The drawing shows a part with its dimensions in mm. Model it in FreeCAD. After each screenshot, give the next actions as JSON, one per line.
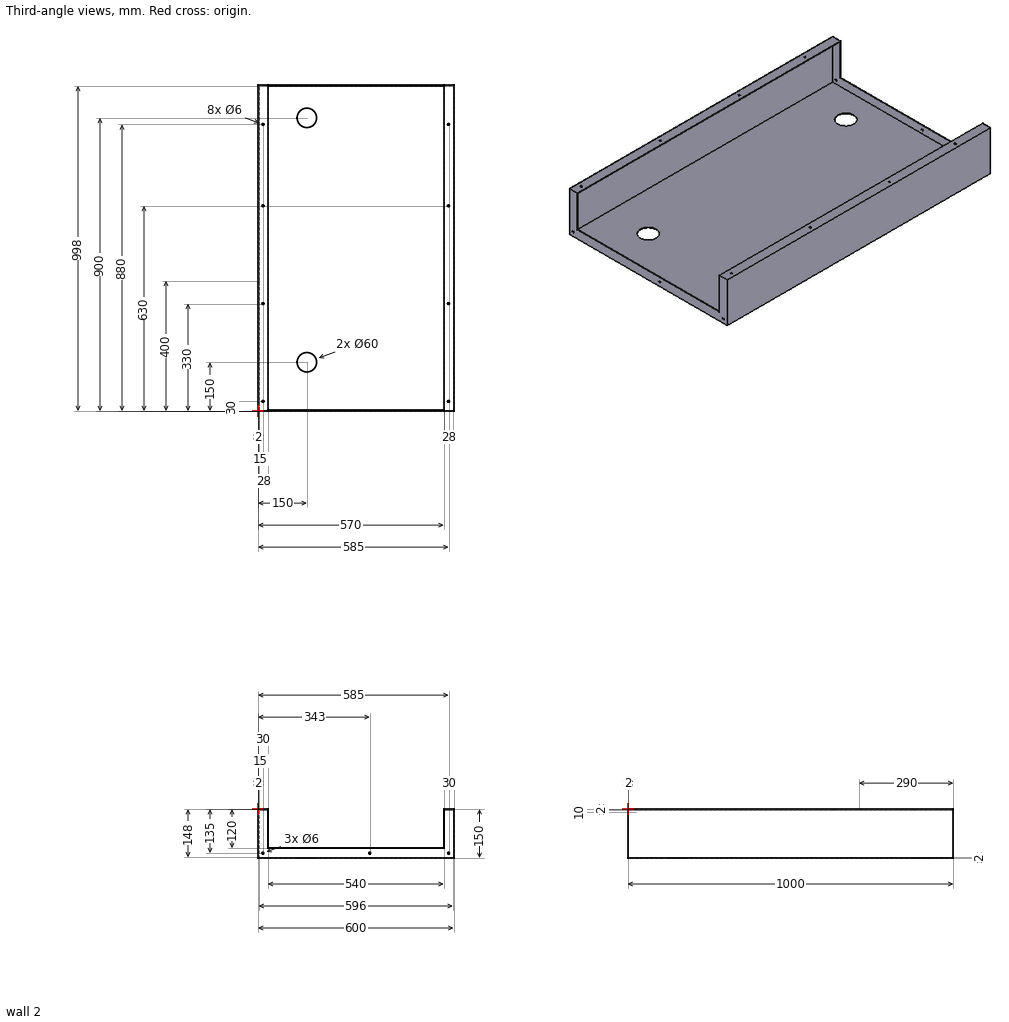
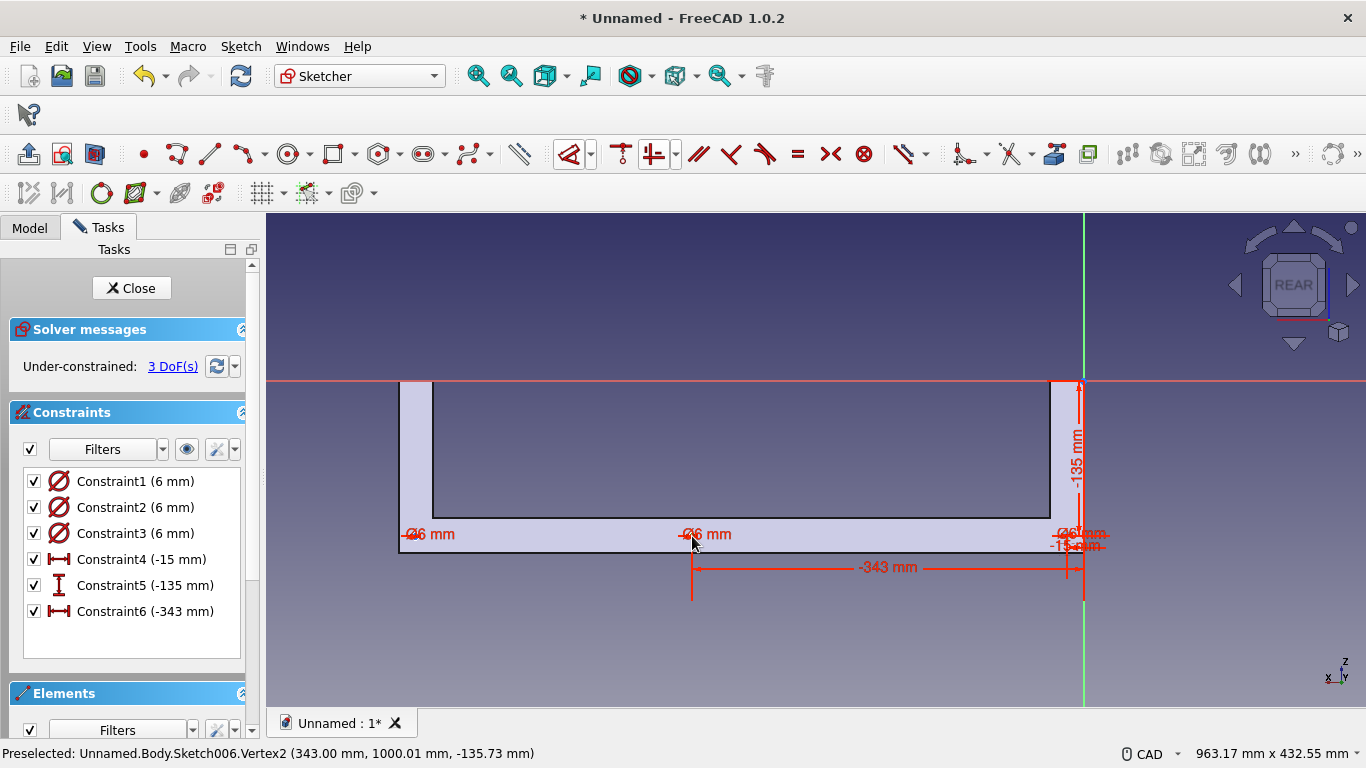
{"action": "key", "text": "i"}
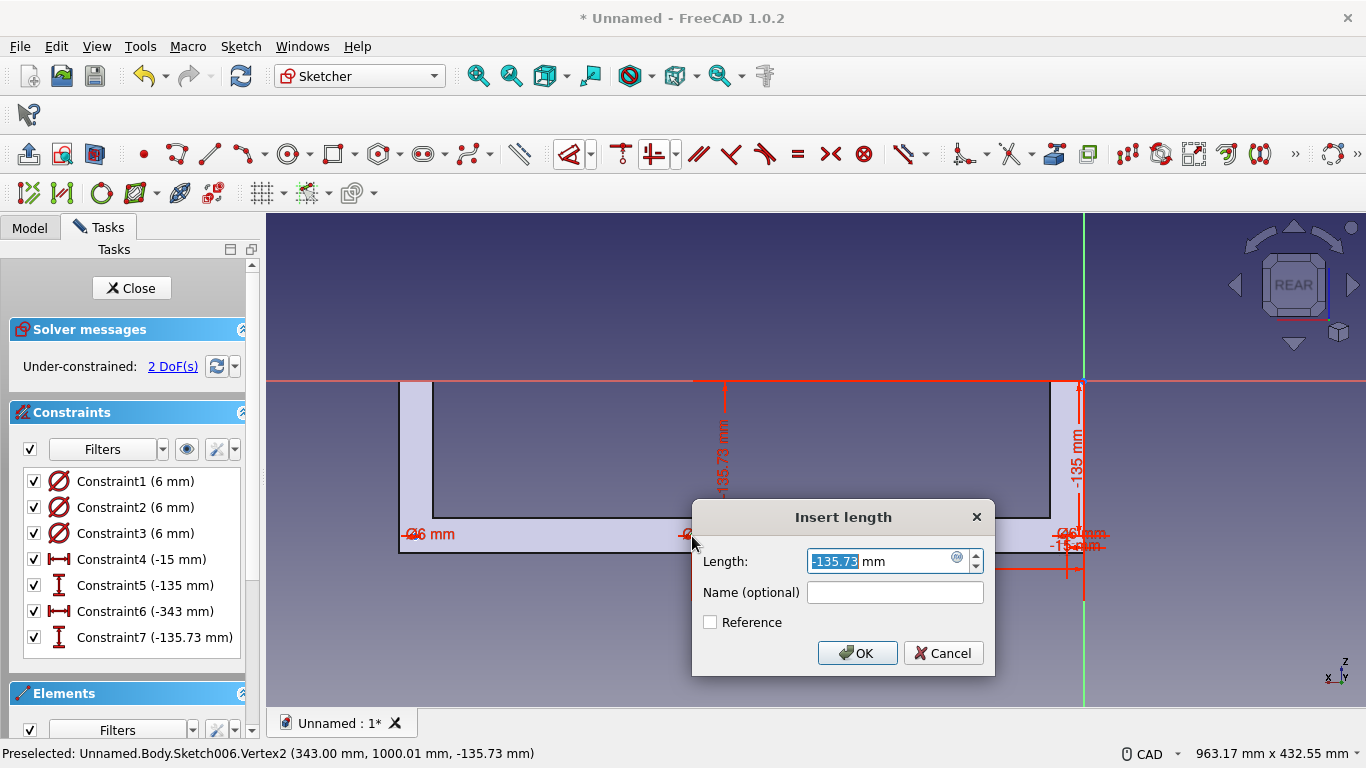
{"action": "type", "text": "-135"}
{"action": "key", "text": "Return"}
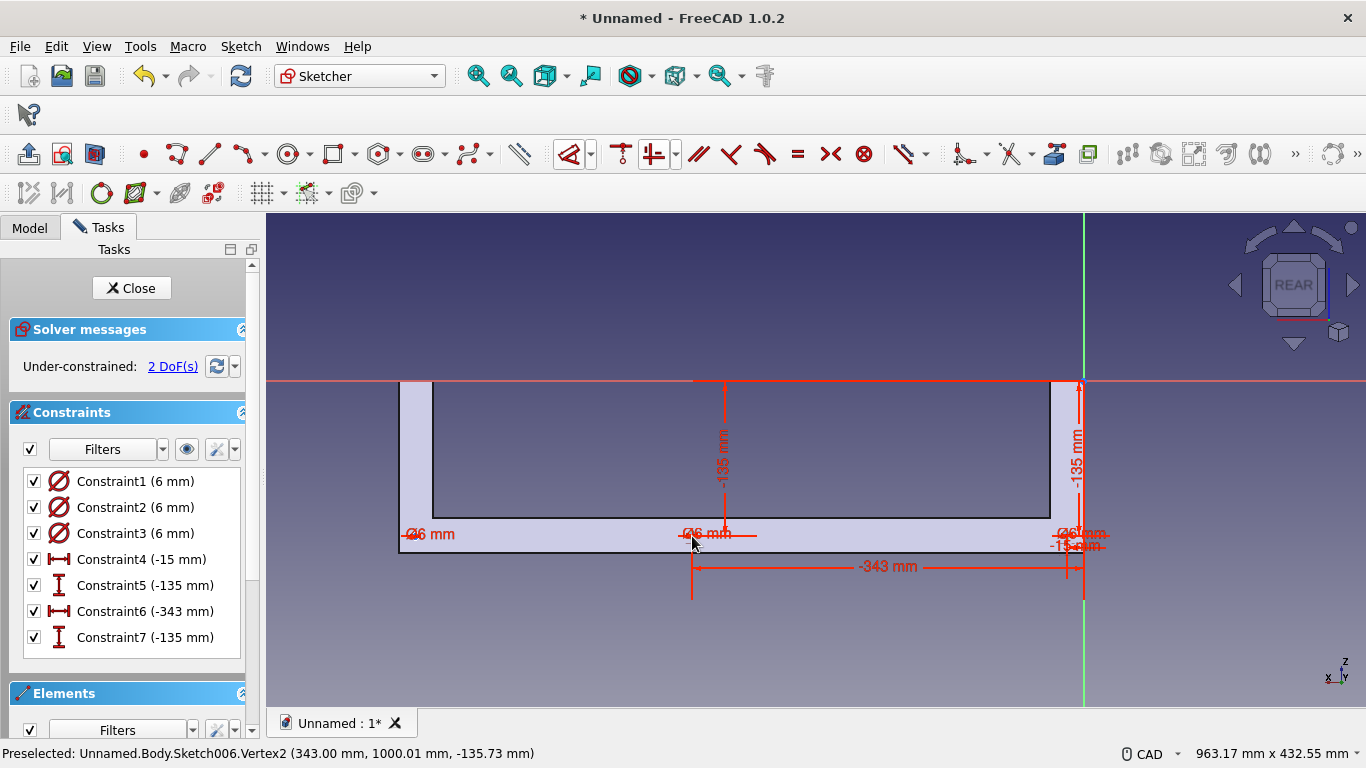
{"action": "left_click", "coordinate": [416, 536]}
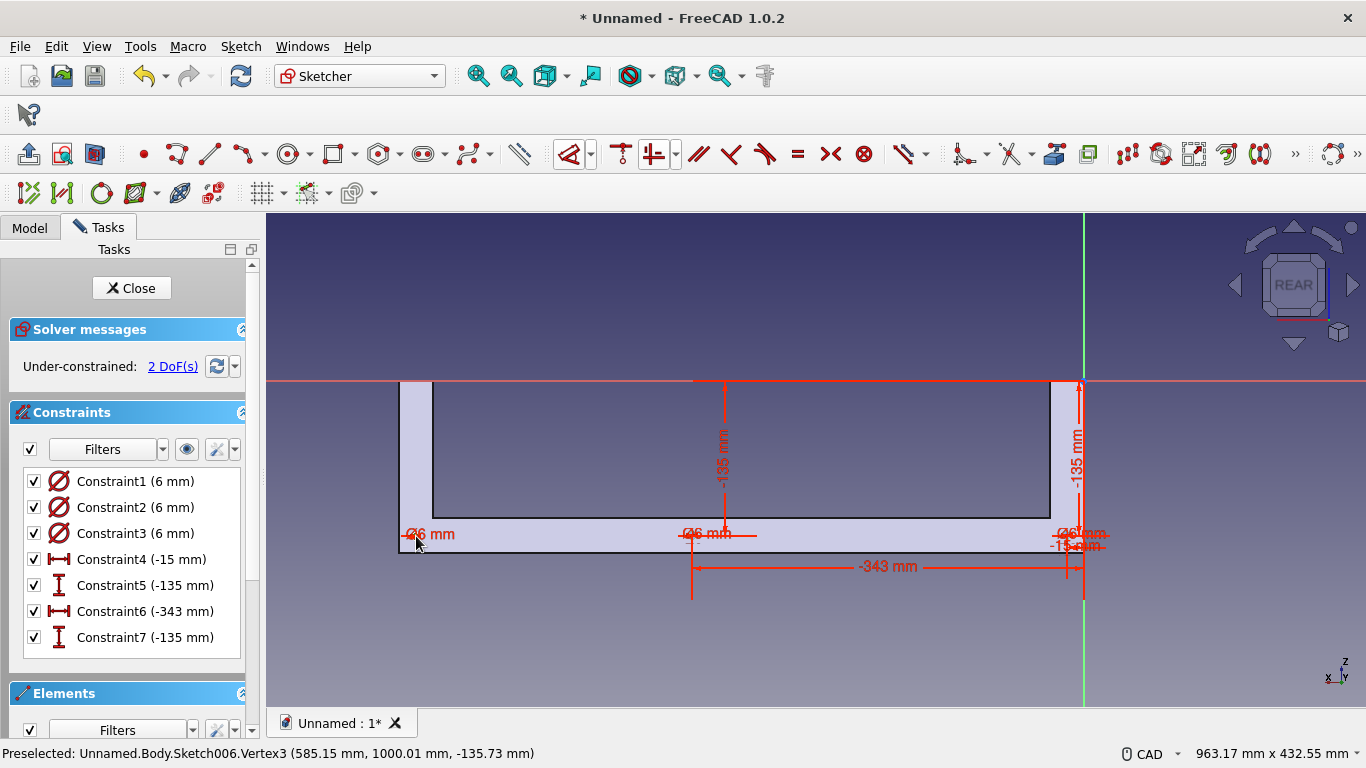
{"action": "left_click", "coordinate": [590, 154]}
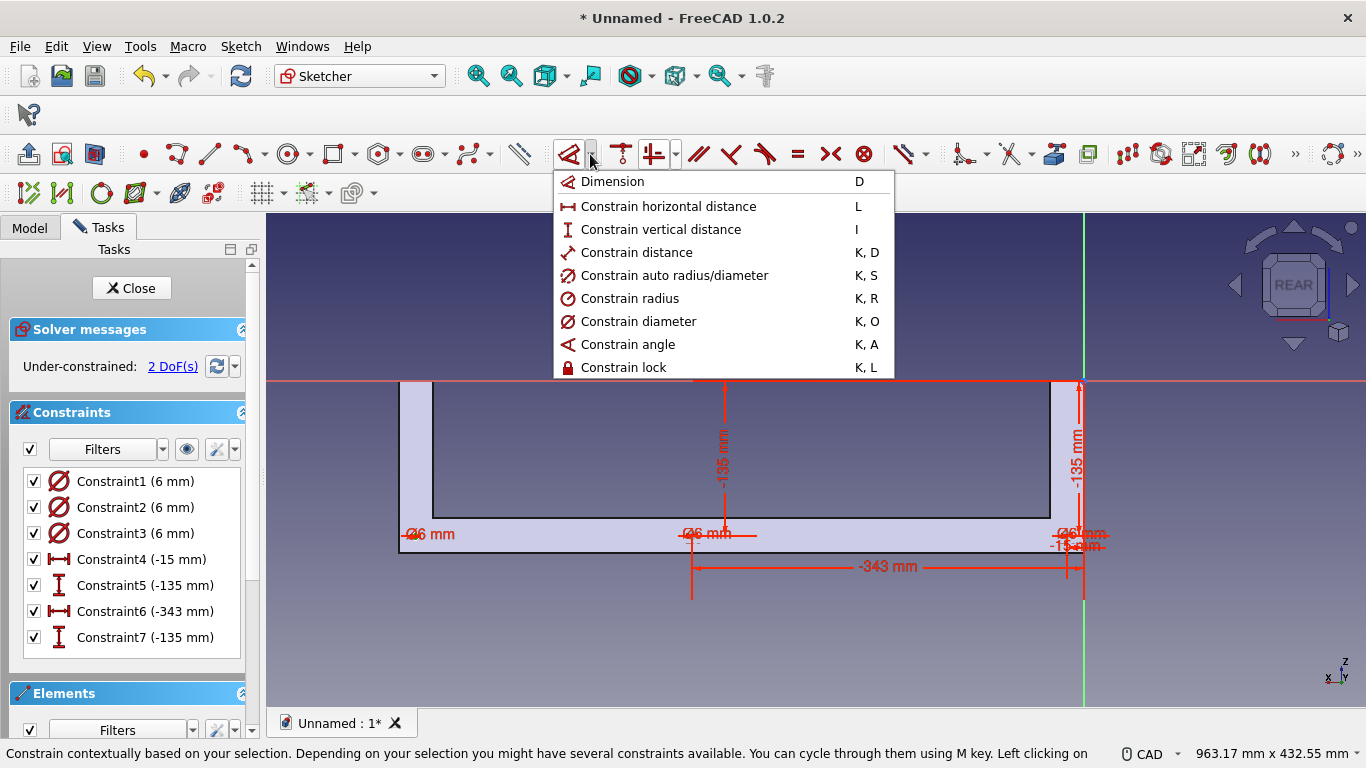
{"action": "left_click", "coordinate": [724, 206]}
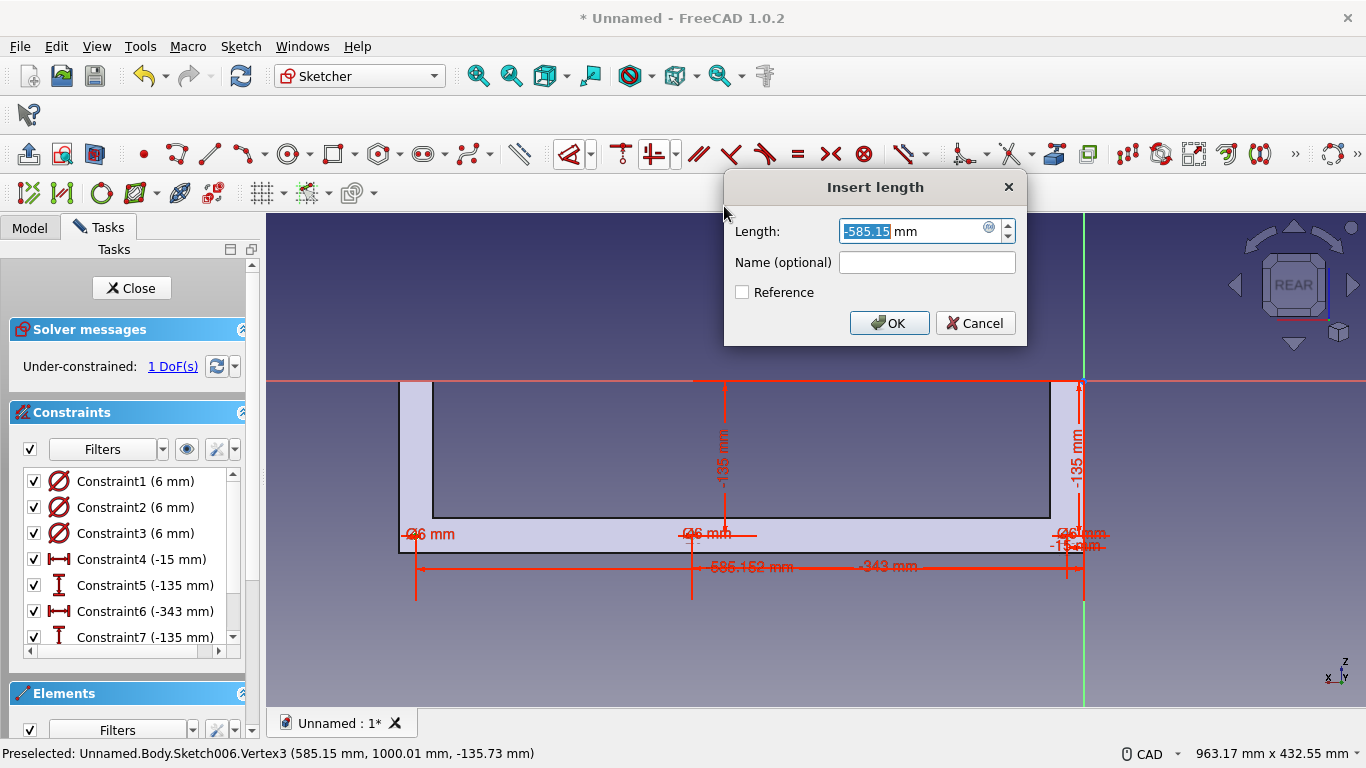
{"action": "type", "text": "-585"}
{"action": "key", "text": "Return"}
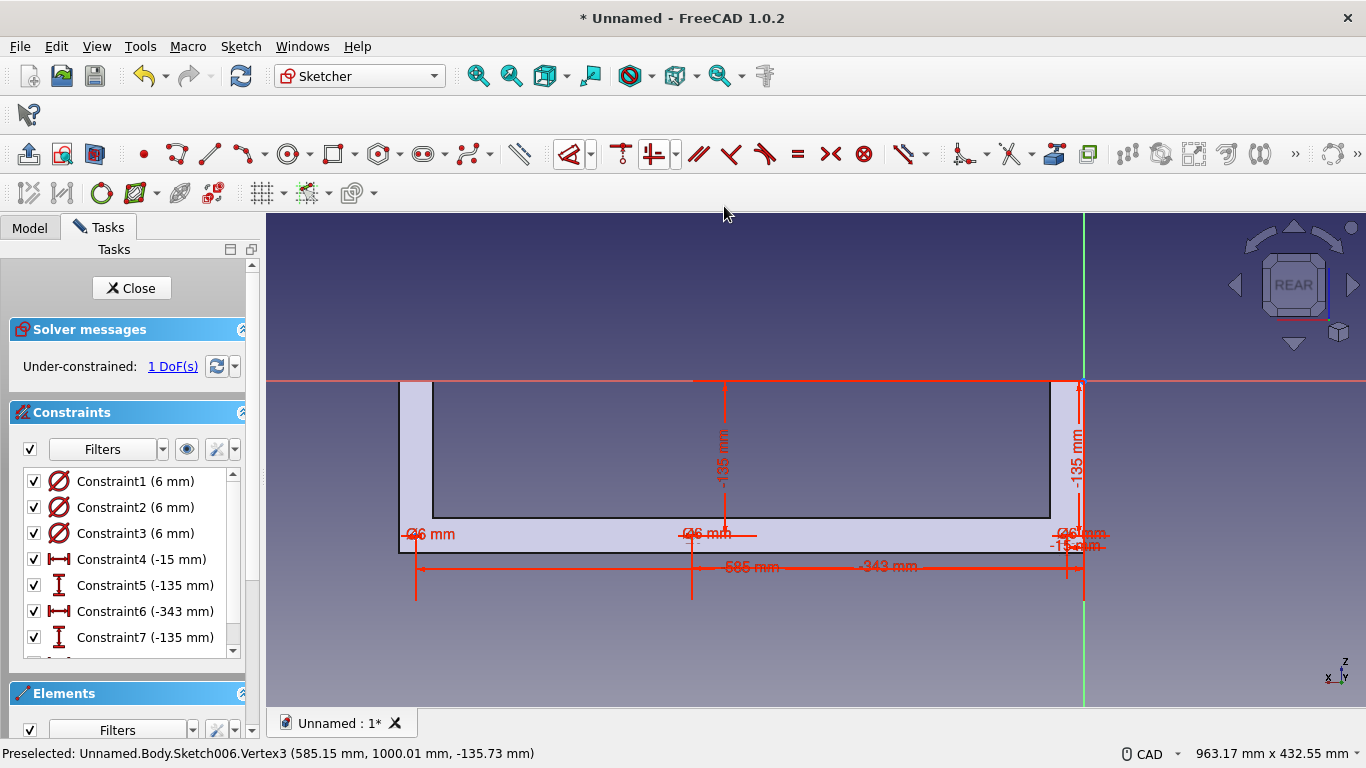
{"action": "left_click", "coordinate": [416, 536]}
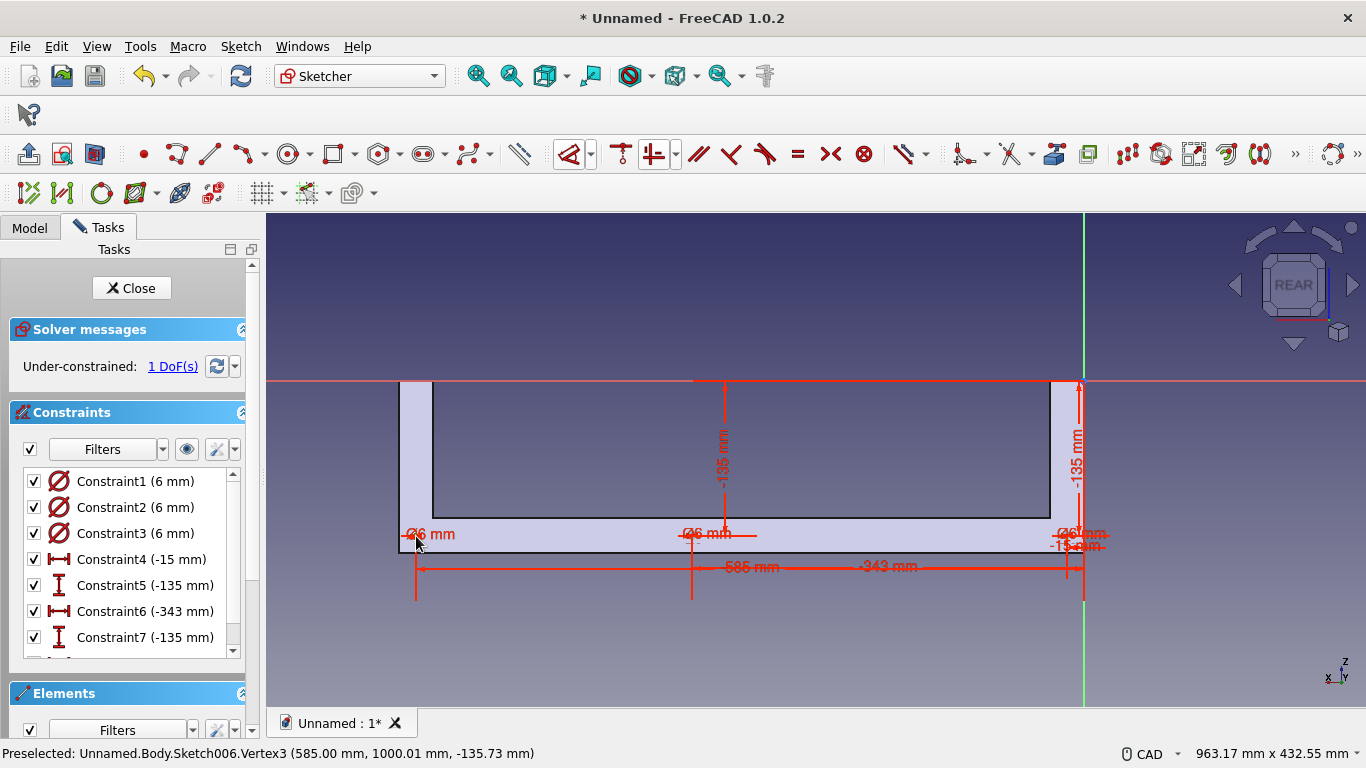
{"action": "left_click", "coordinate": [590, 154]}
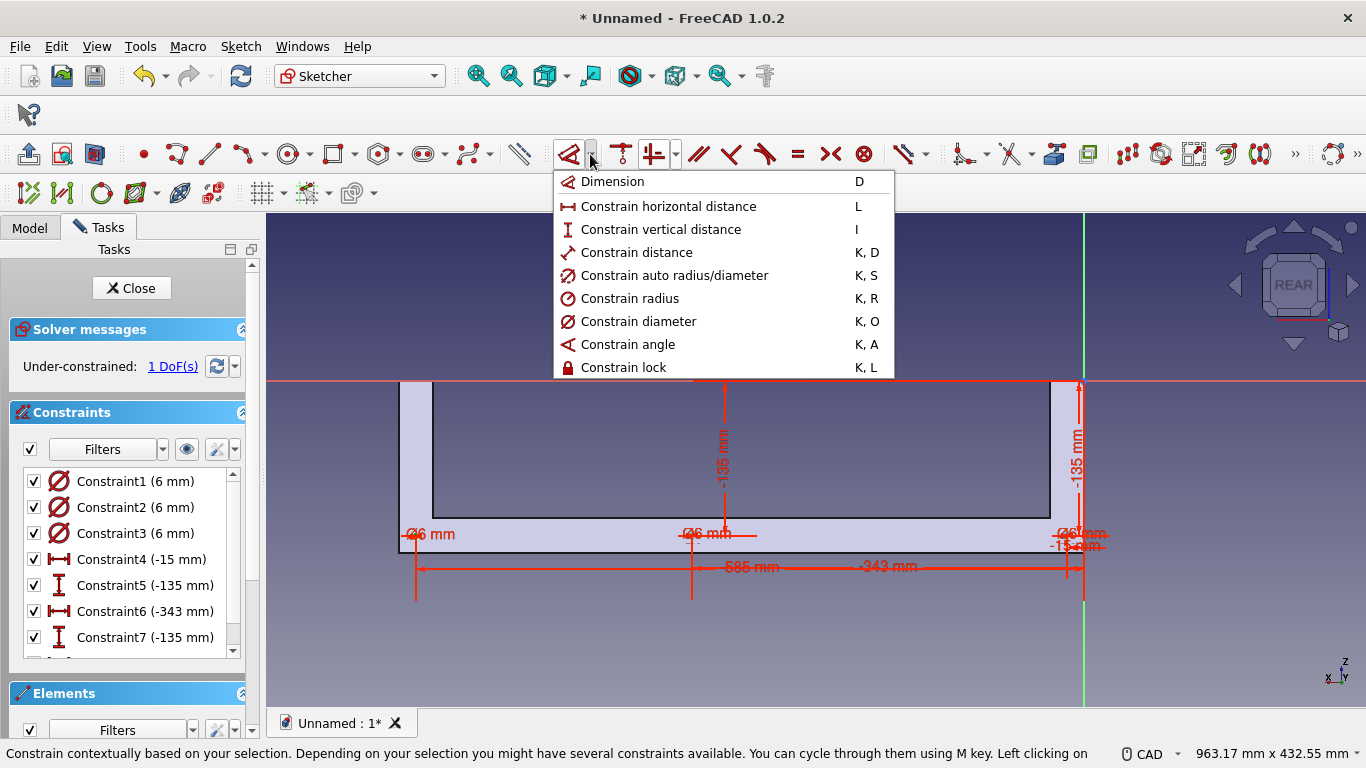
{"action": "left_click", "coordinate": [724, 230]}